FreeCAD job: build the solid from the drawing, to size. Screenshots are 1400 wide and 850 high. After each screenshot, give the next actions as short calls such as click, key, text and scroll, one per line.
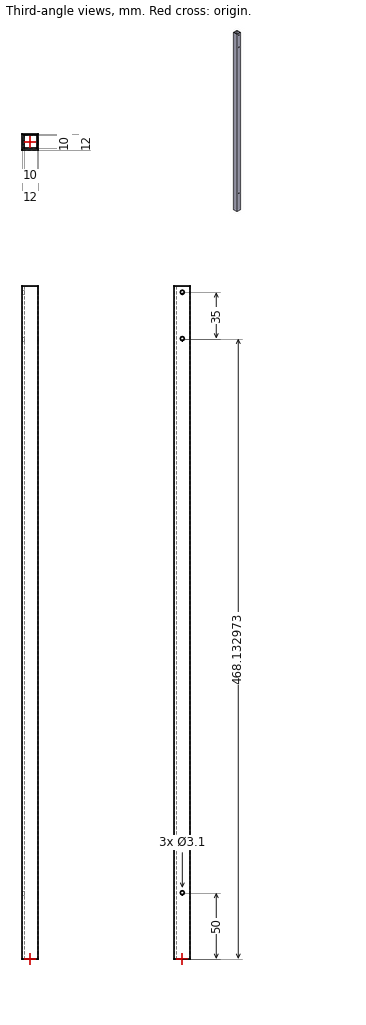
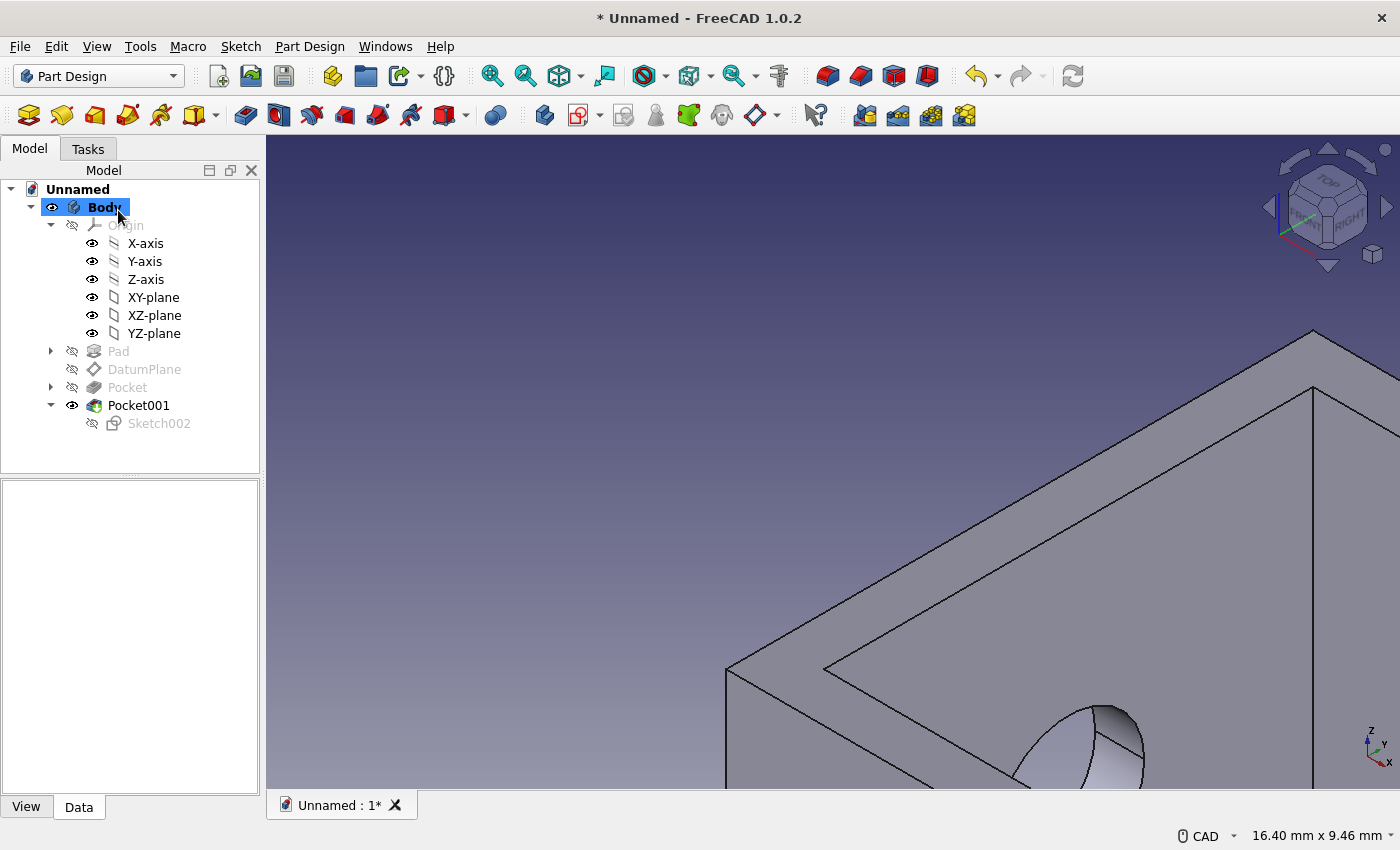
click(493, 76)